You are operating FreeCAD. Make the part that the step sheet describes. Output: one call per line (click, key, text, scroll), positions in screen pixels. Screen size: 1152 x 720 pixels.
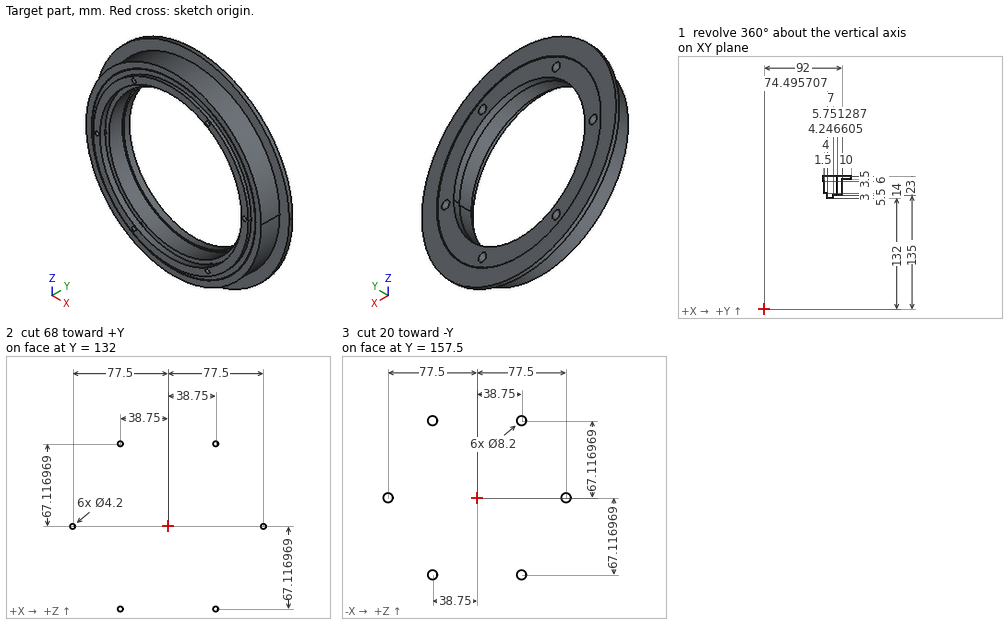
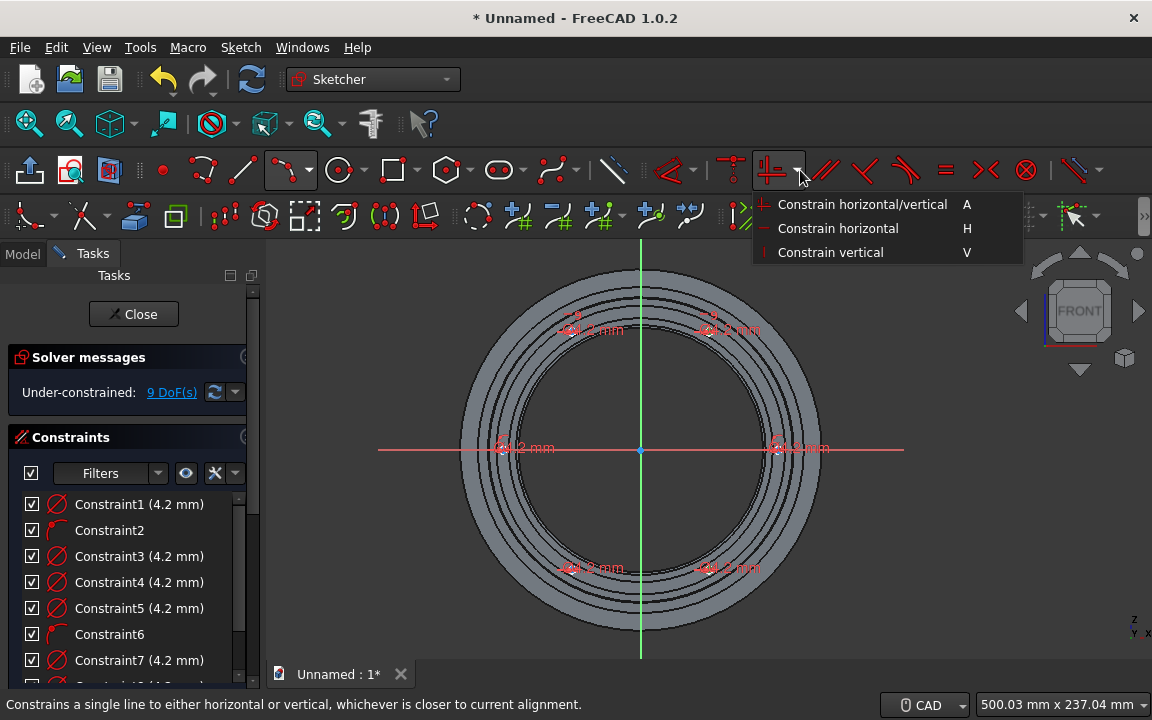
click(888, 252)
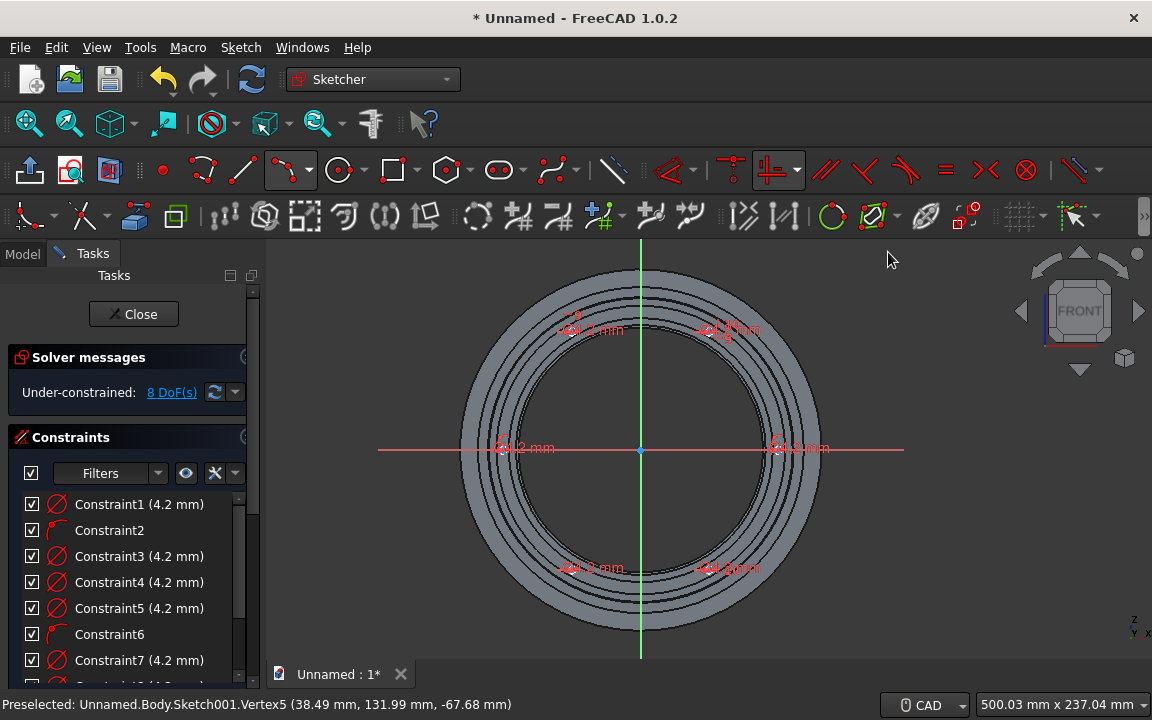
click(572, 332)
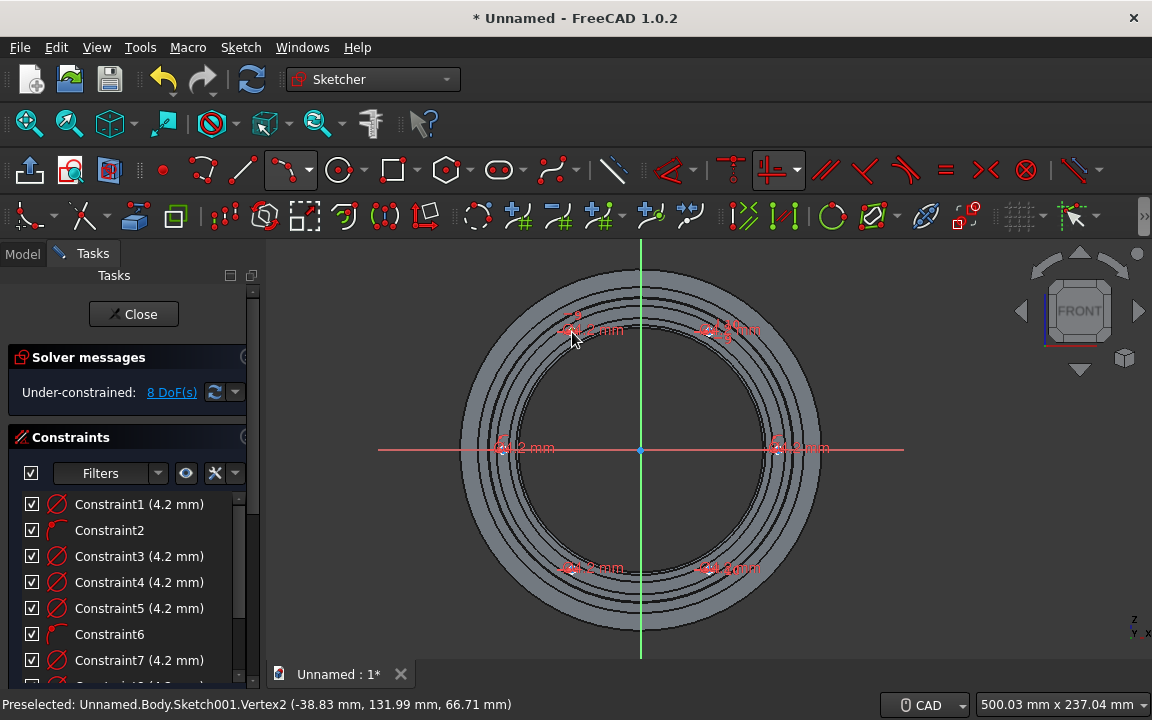
click(572, 570)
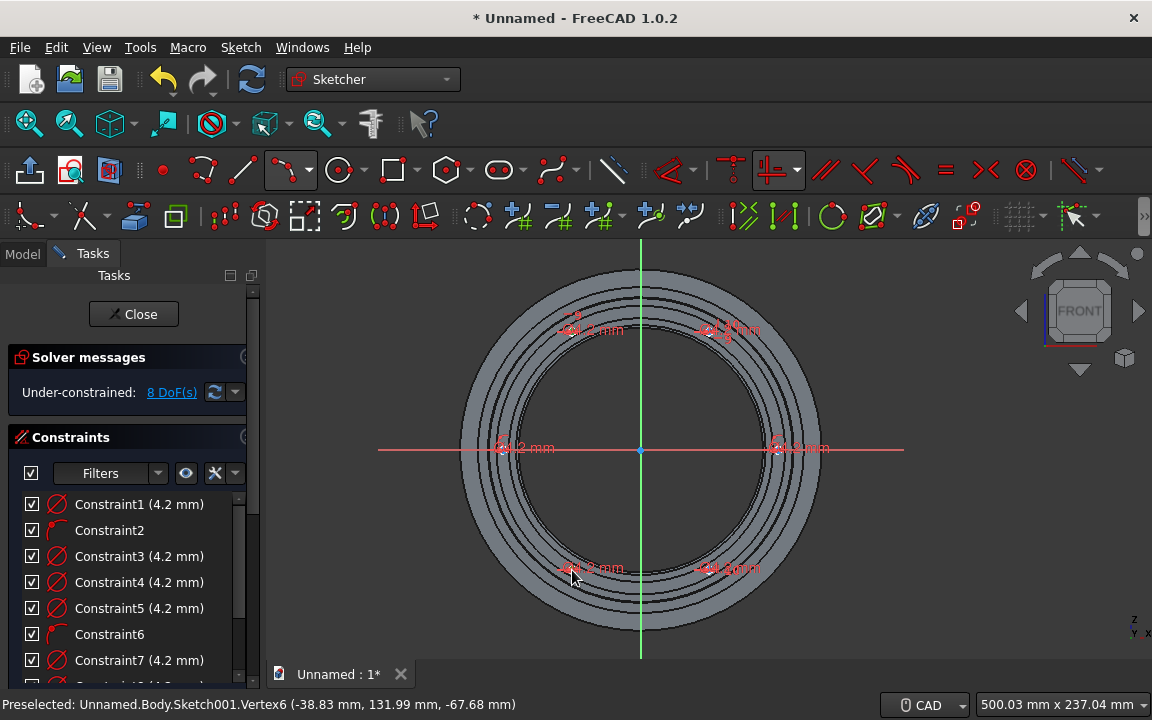
click(800, 170)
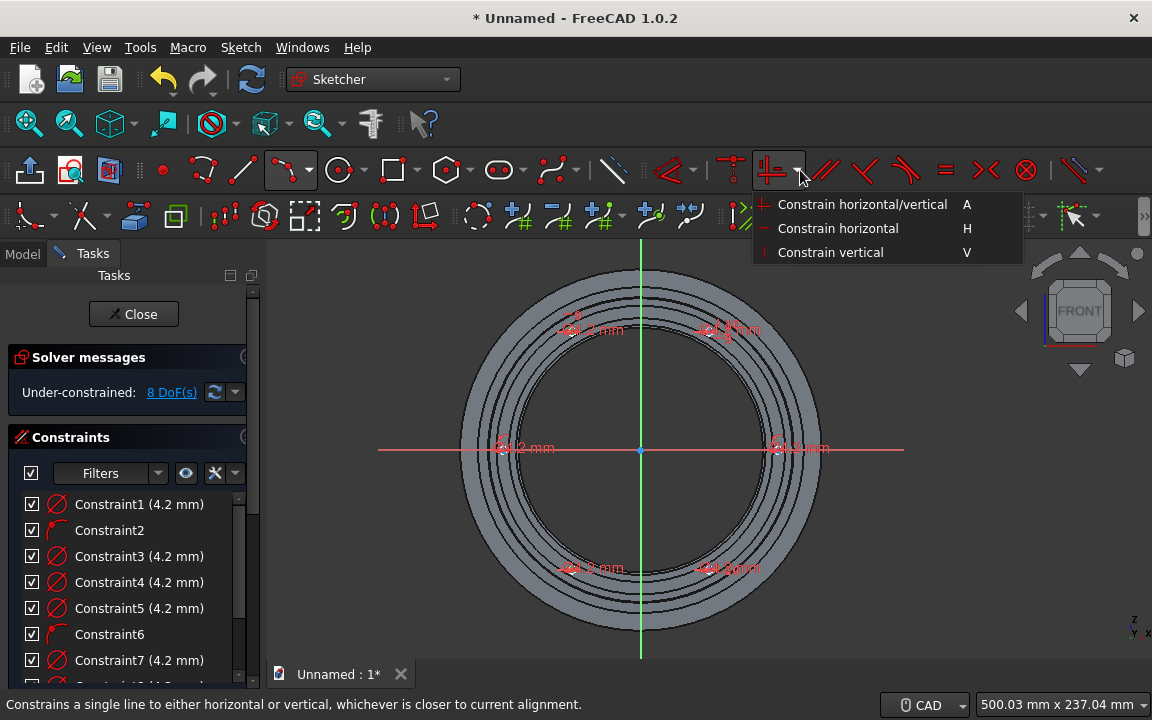
click(888, 252)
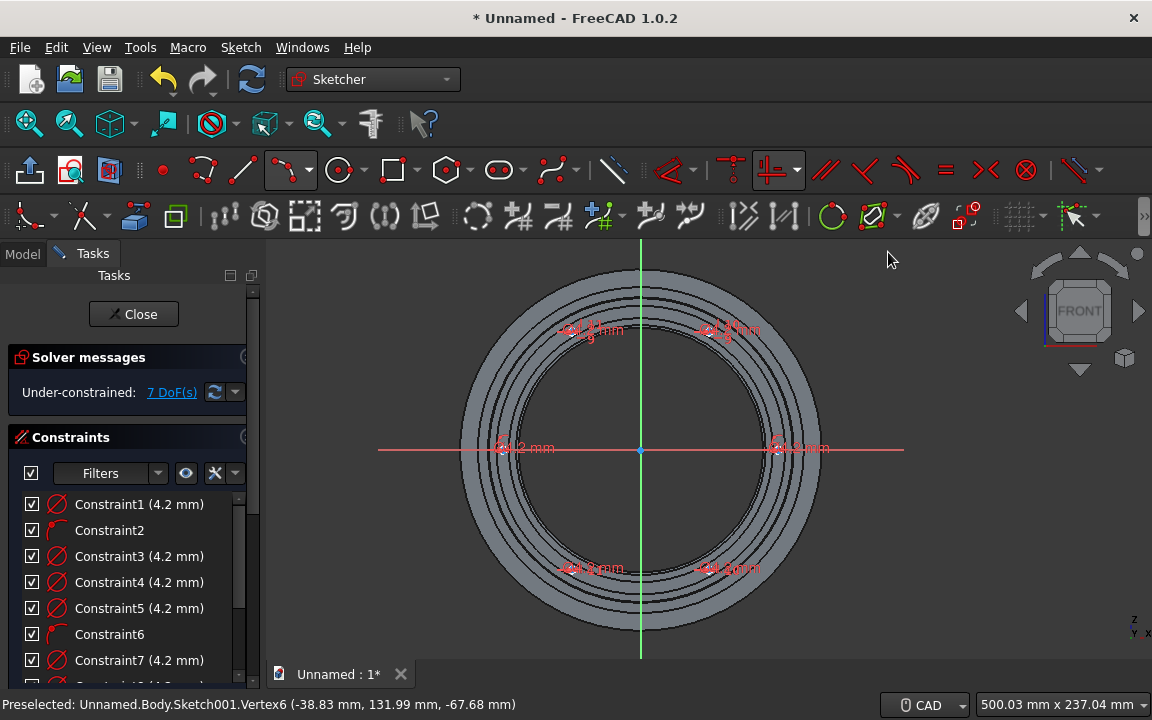
click(709, 570)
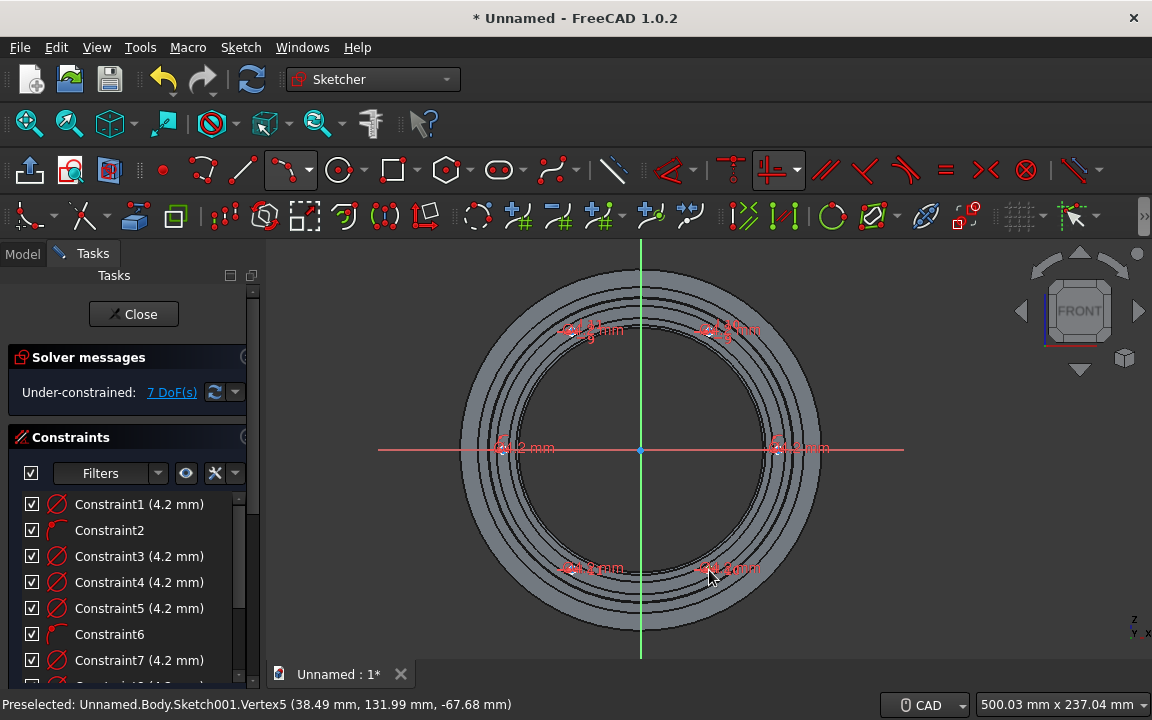
click(572, 570)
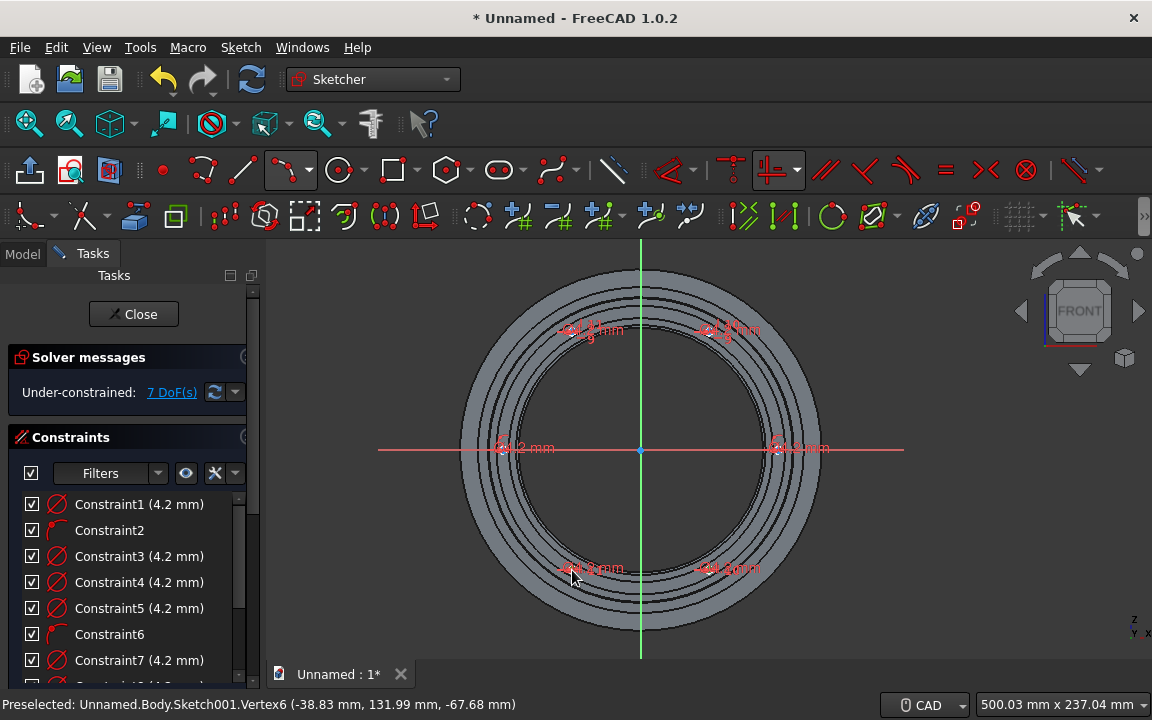
click(800, 170)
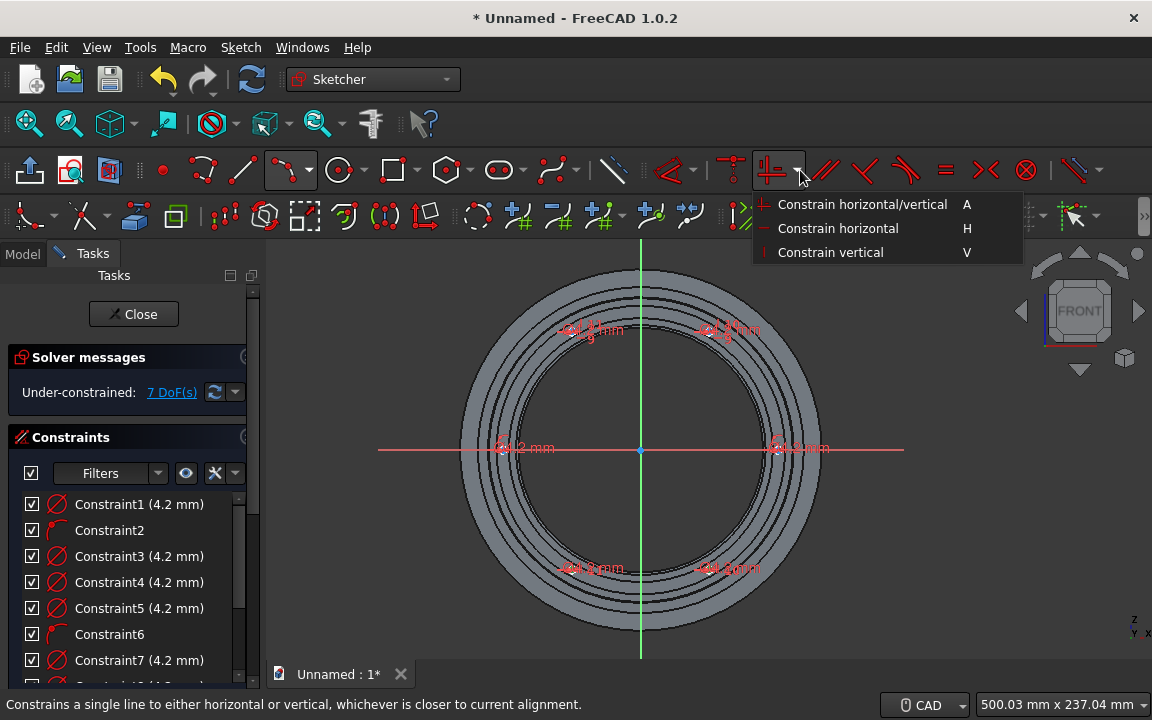
click(888, 228)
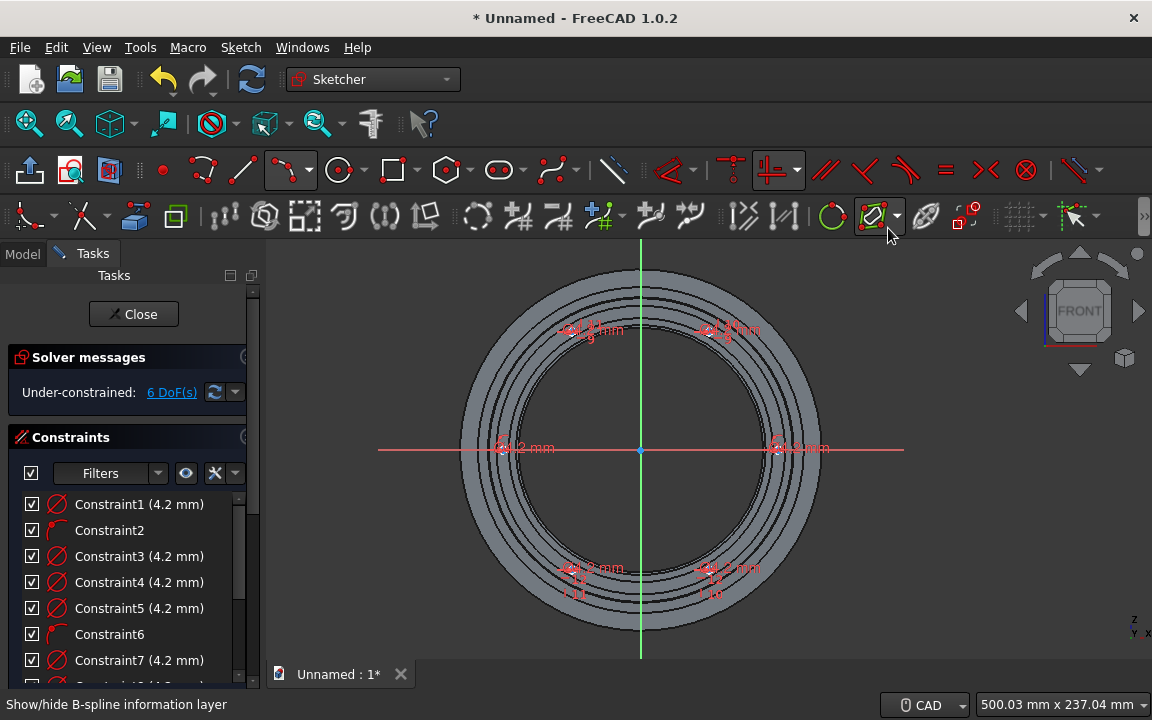
click(668, 170)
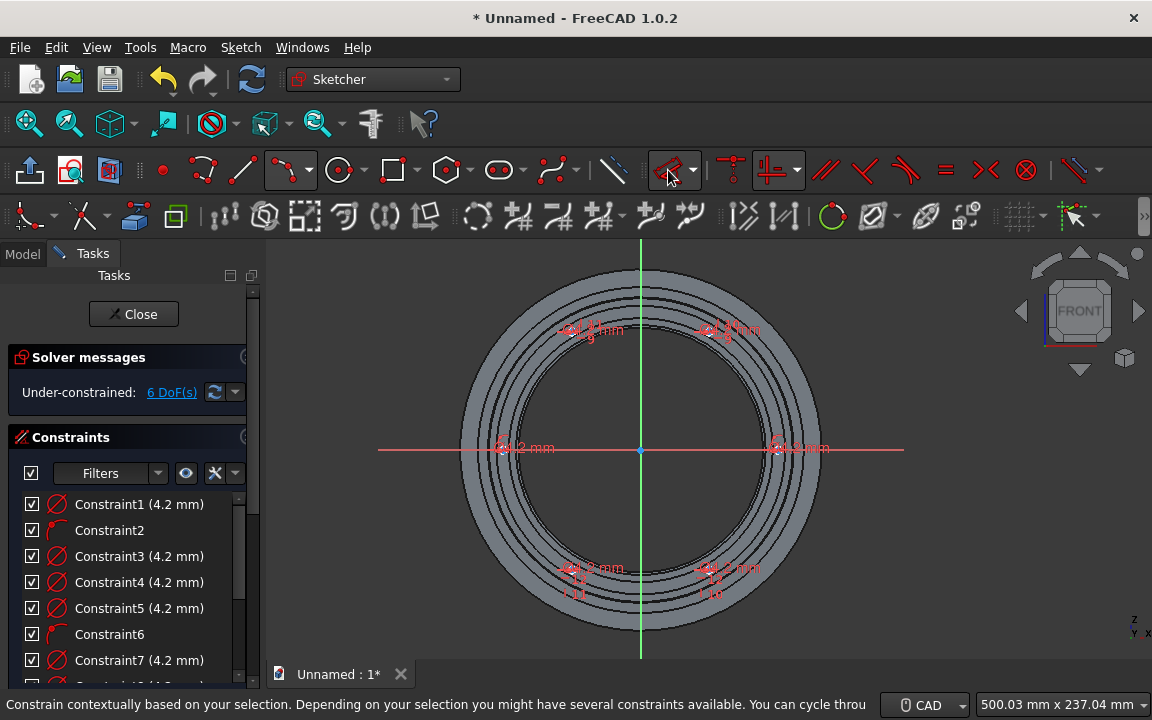
click(503, 450)
click(572, 484)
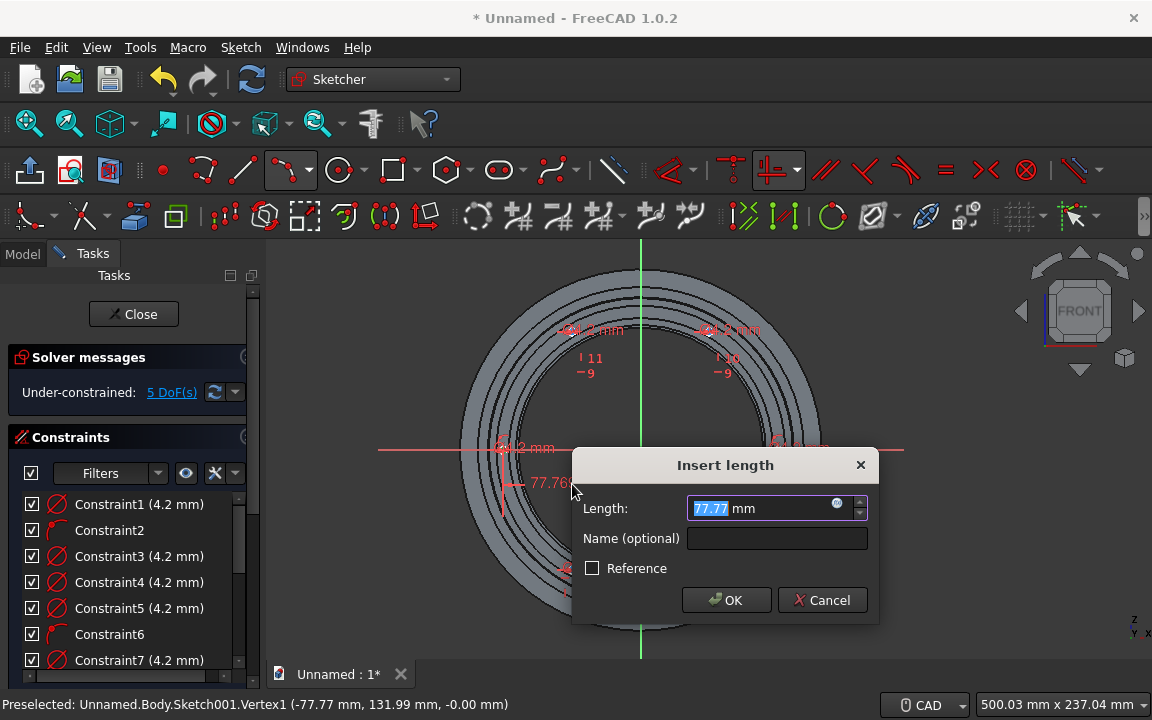
text(77.5)
key(Return)